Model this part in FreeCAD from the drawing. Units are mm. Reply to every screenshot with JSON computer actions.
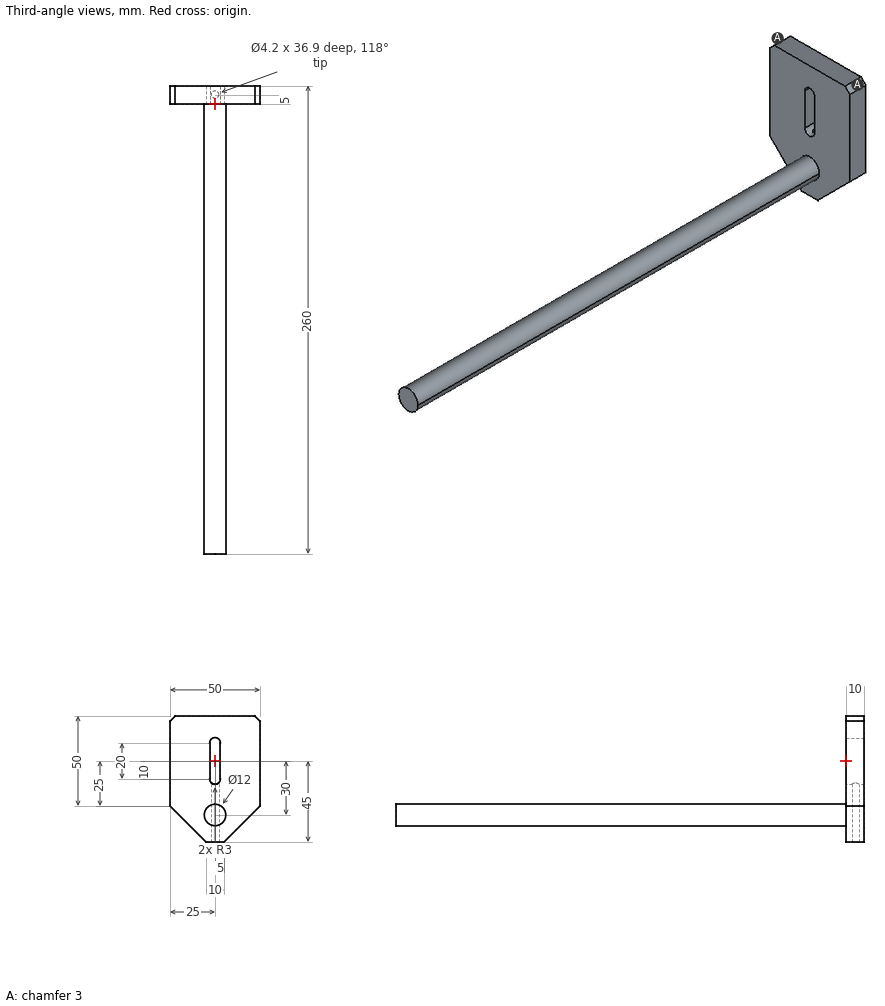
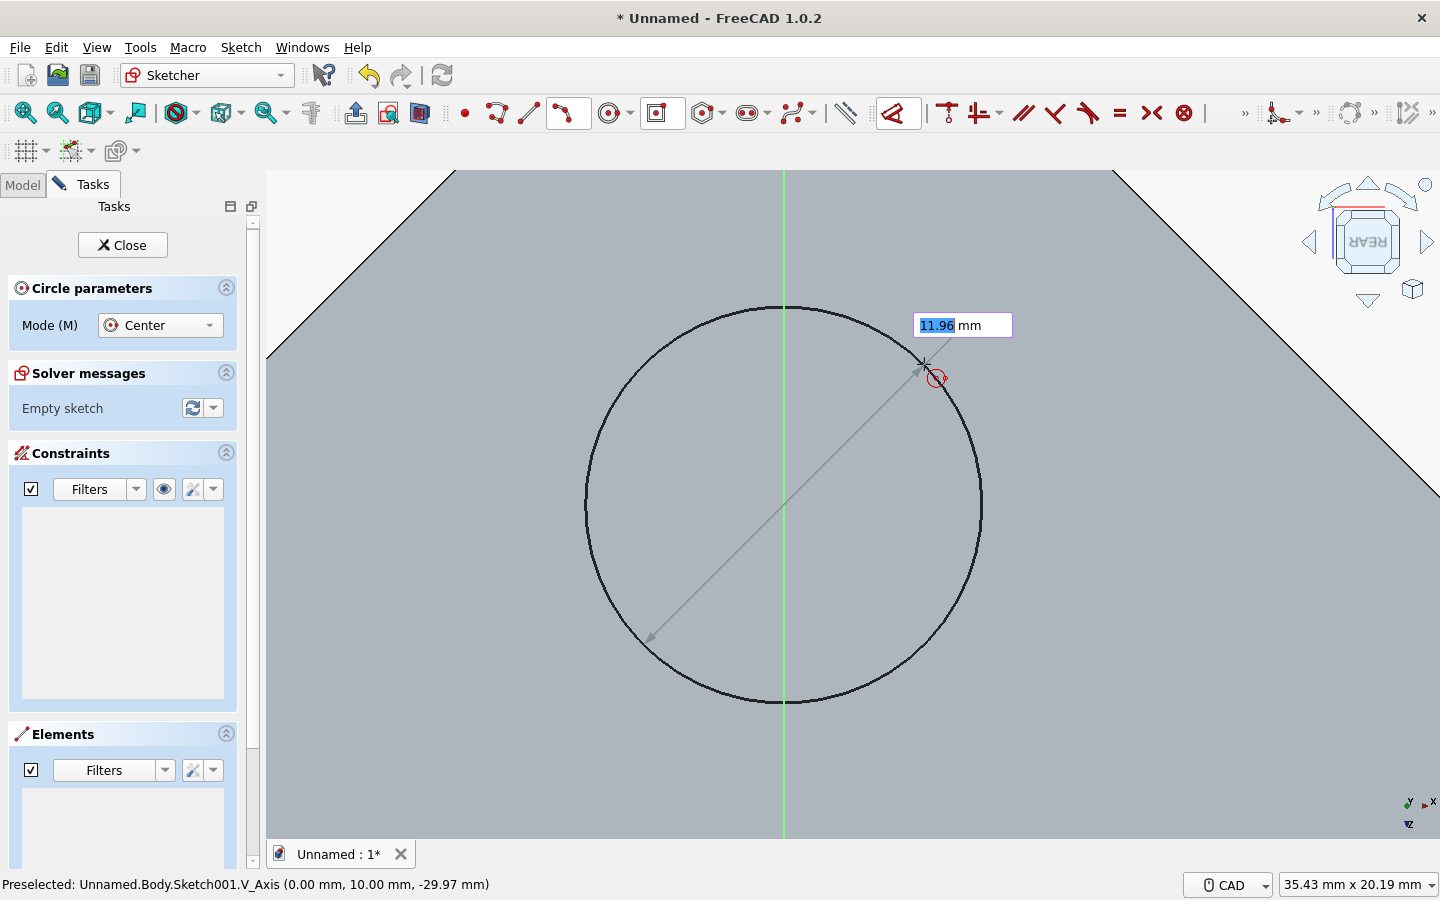
{"action": "type", "text": "12"}
{"action": "key", "text": "Return"}
{"action": "key", "text": "Escape"}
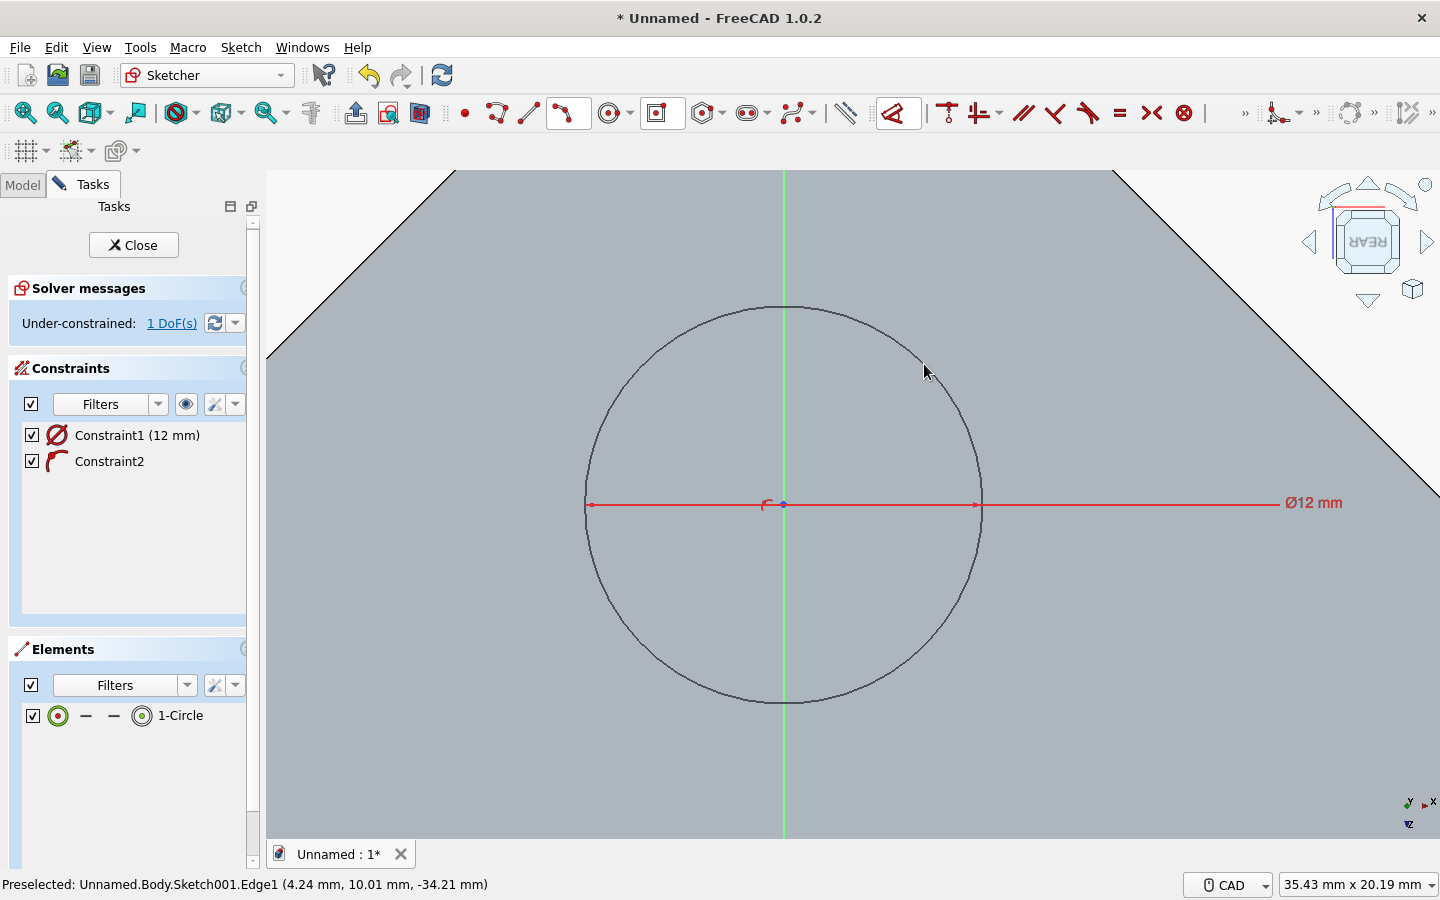
{"action": "left_click", "coordinate": [784, 505]}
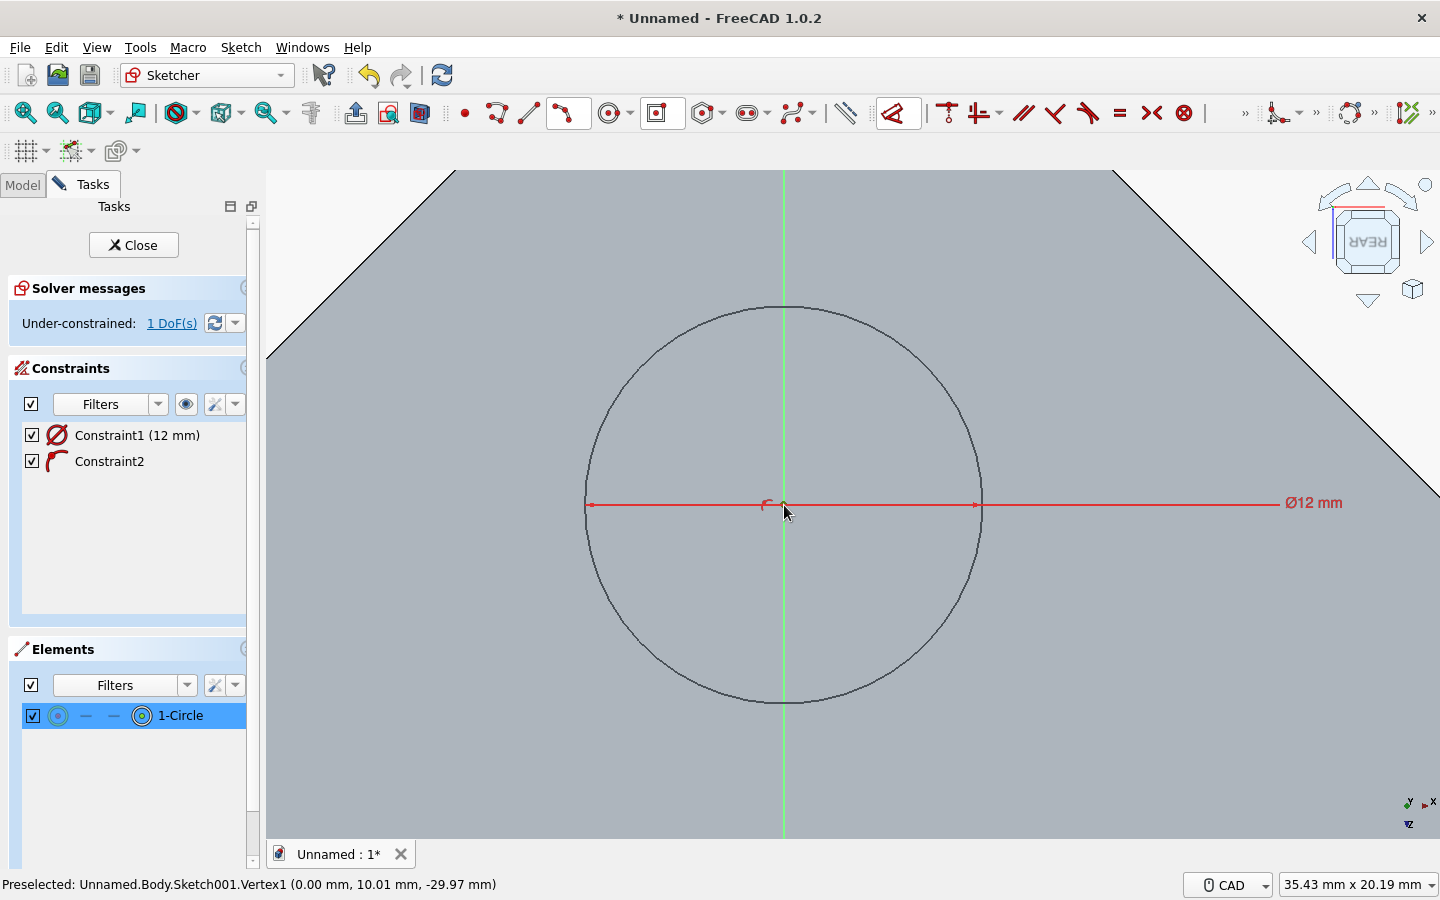
{"action": "key", "text": "i"}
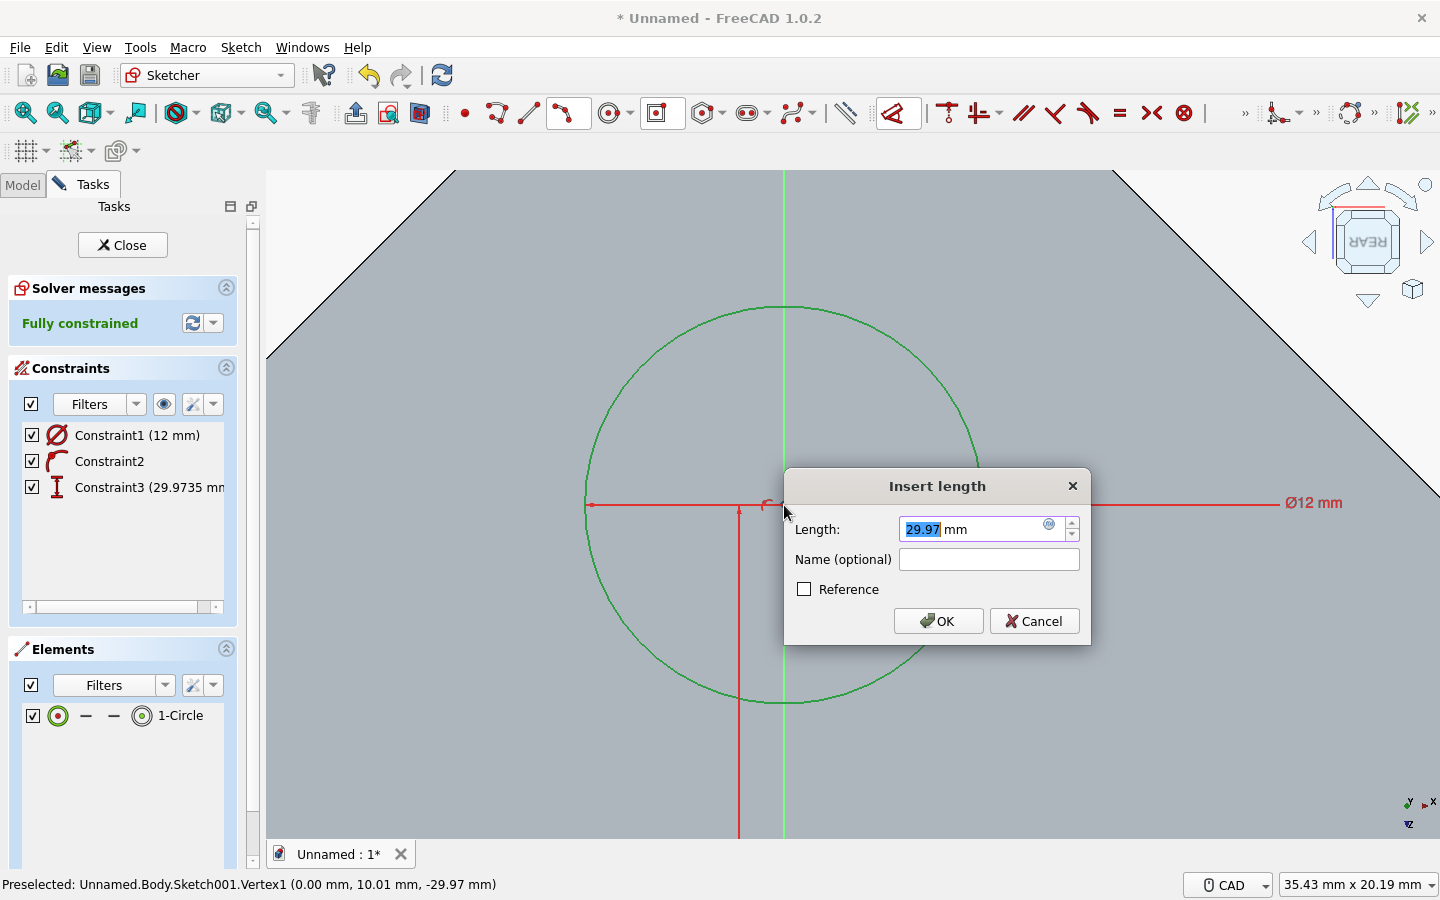
{"action": "type", "text": "30"}
{"action": "key", "text": "Return"}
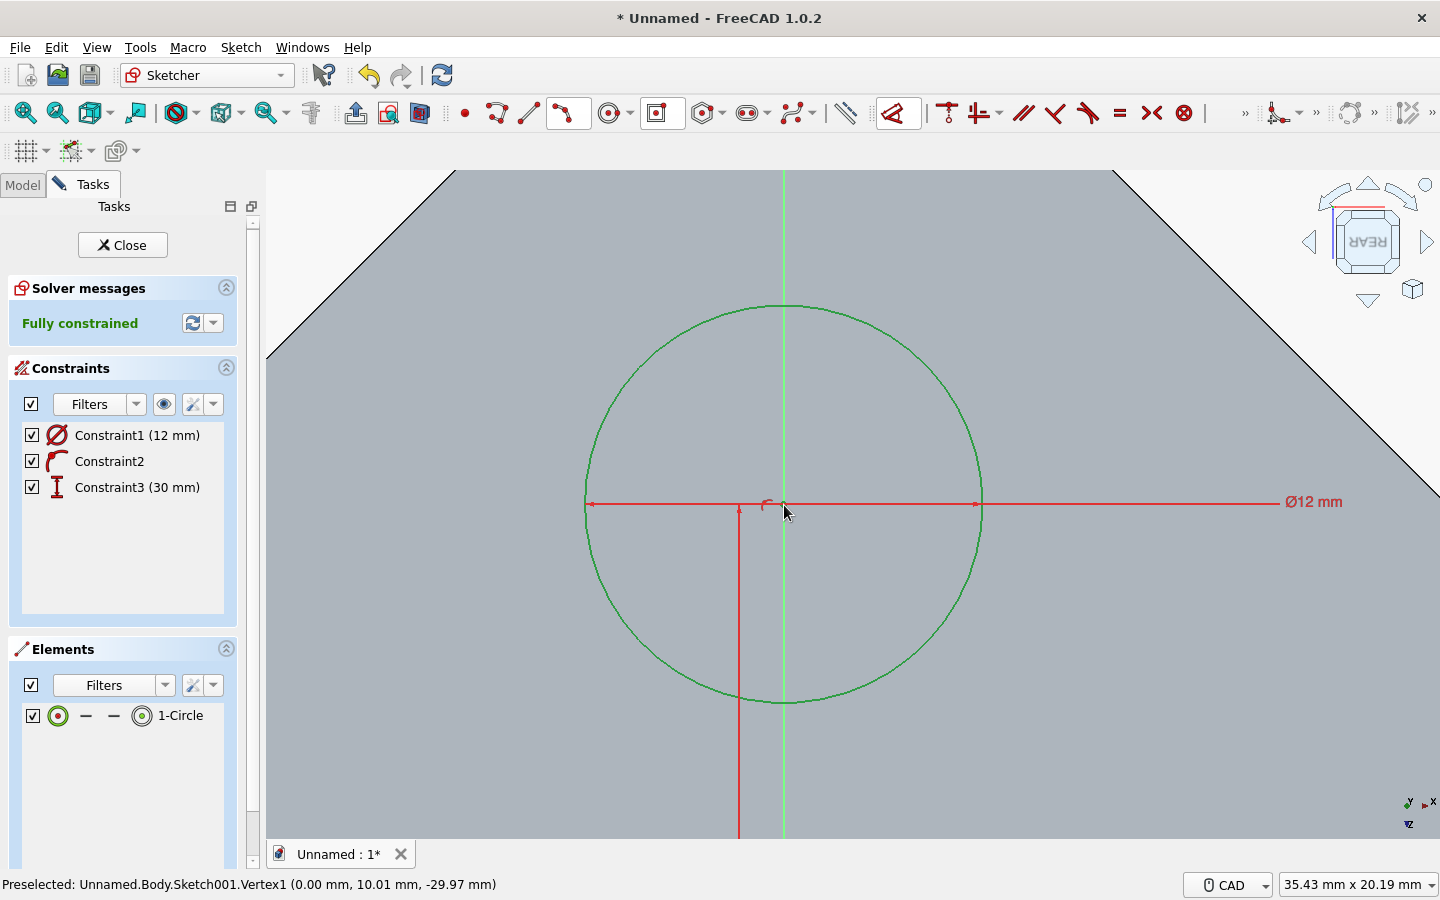
{"action": "left_click", "coordinate": [123, 245]}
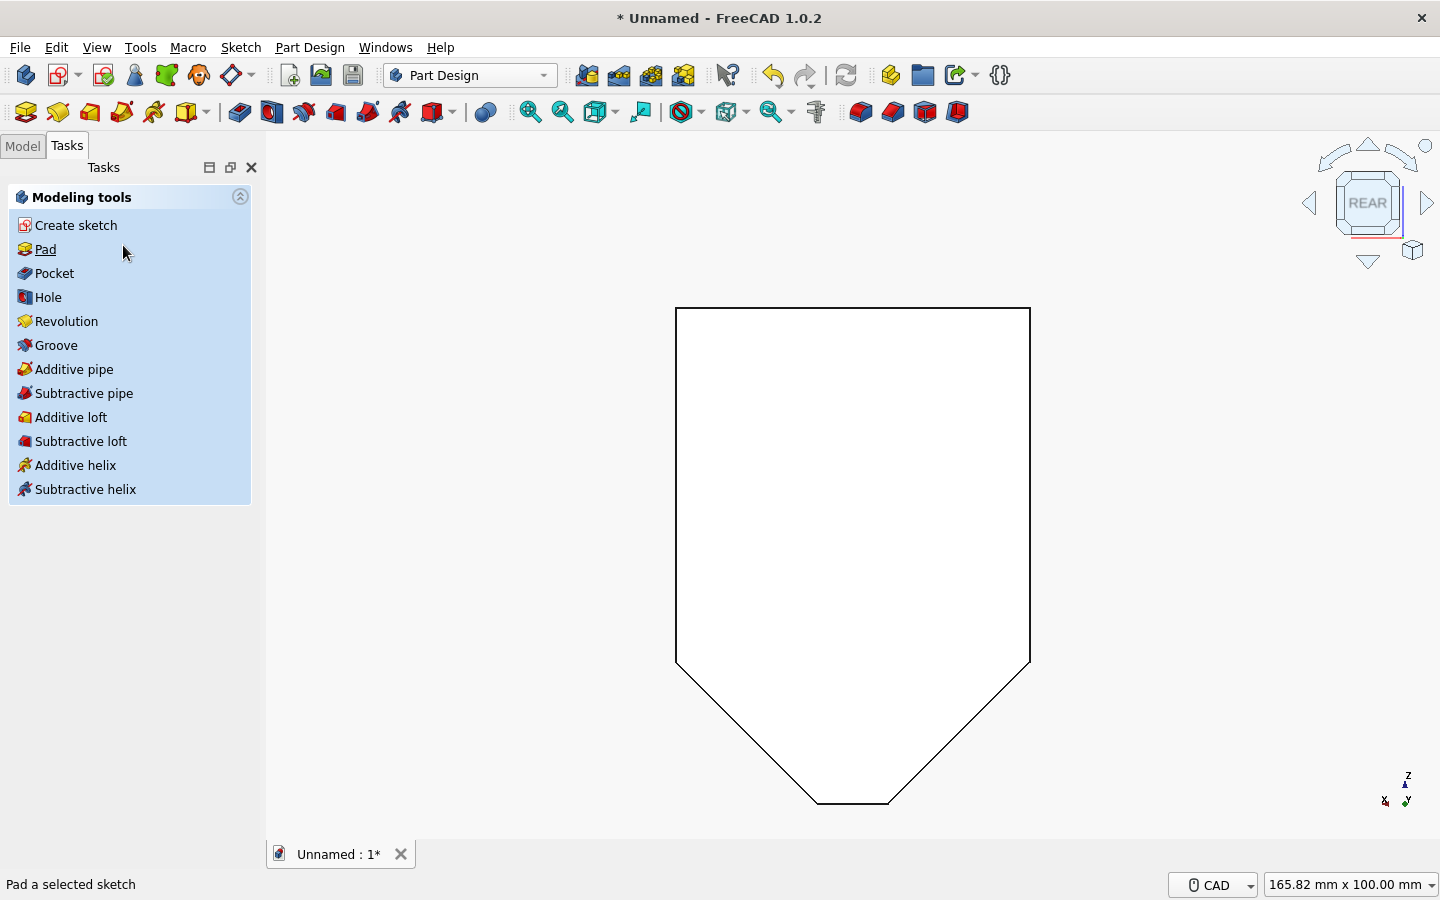
{"action": "left_click", "coordinate": [26, 112]}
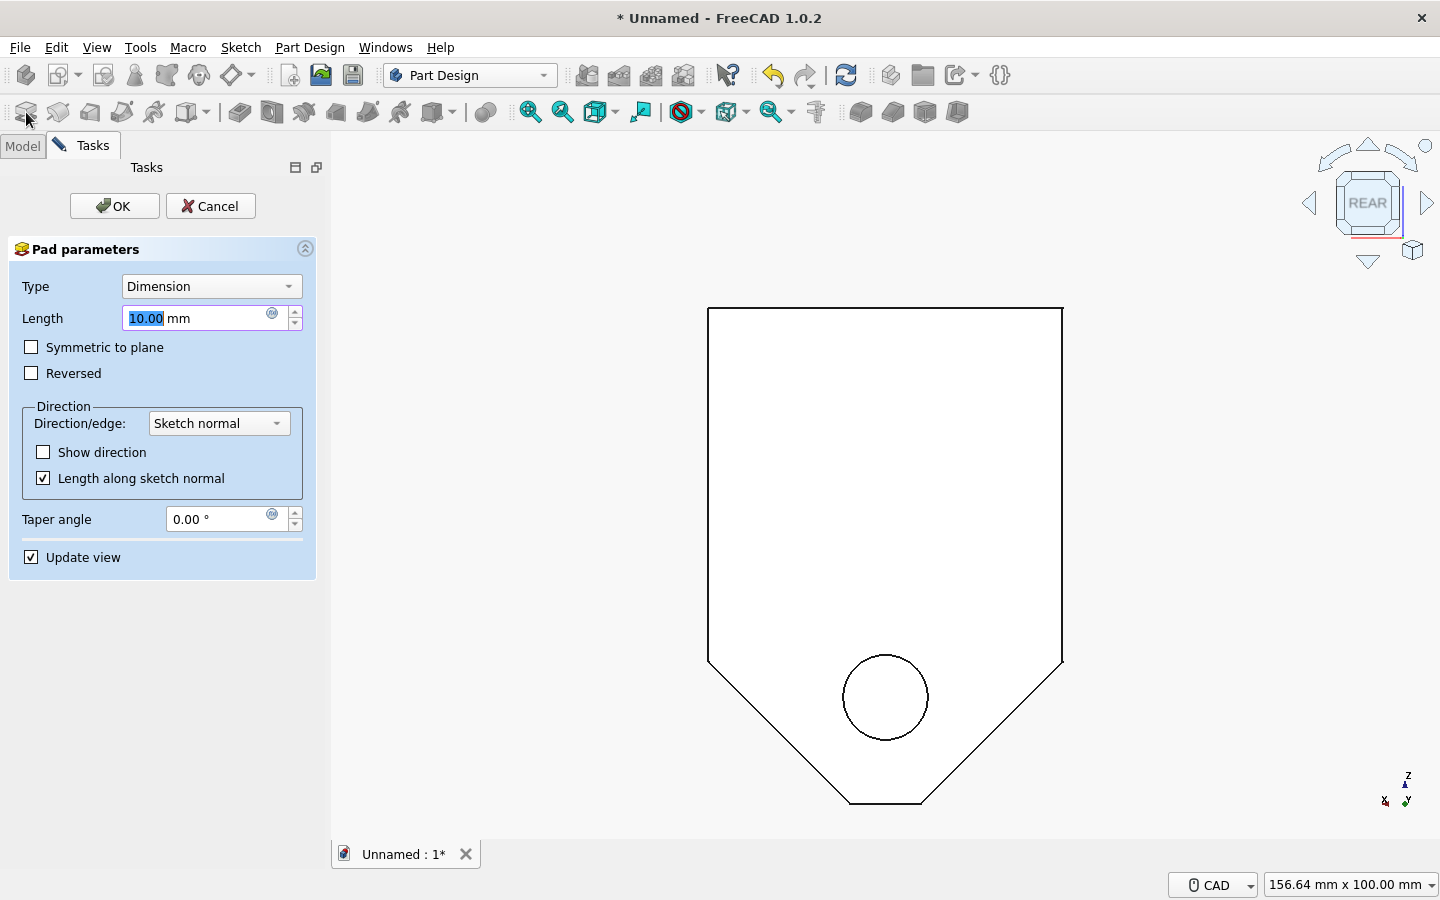
{"action": "type", "text": "260"}
{"action": "key", "text": "Tab"}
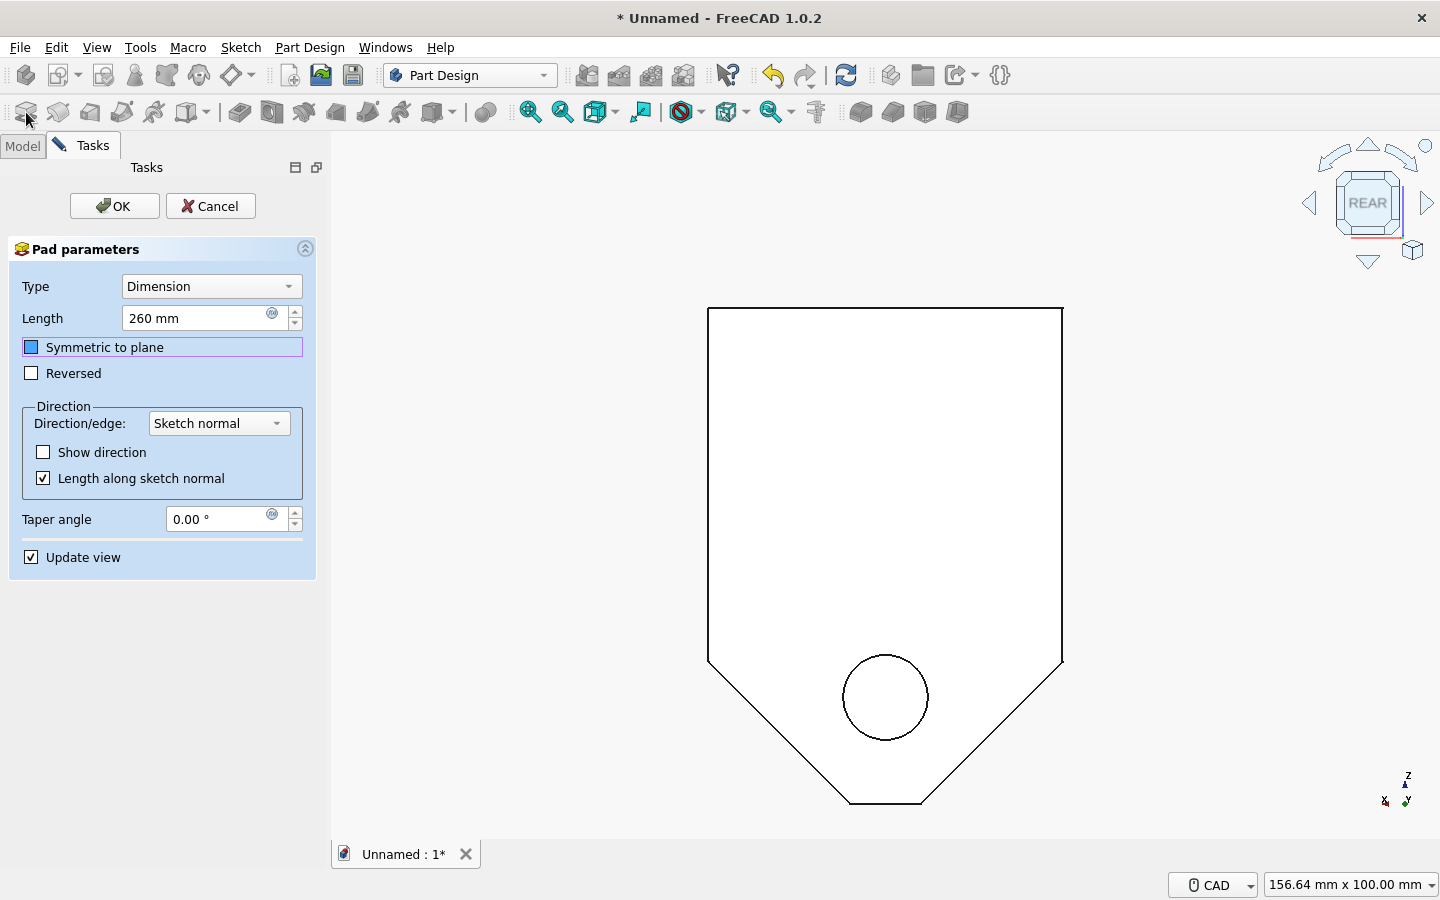
{"action": "left_click", "coordinate": [30, 373]}